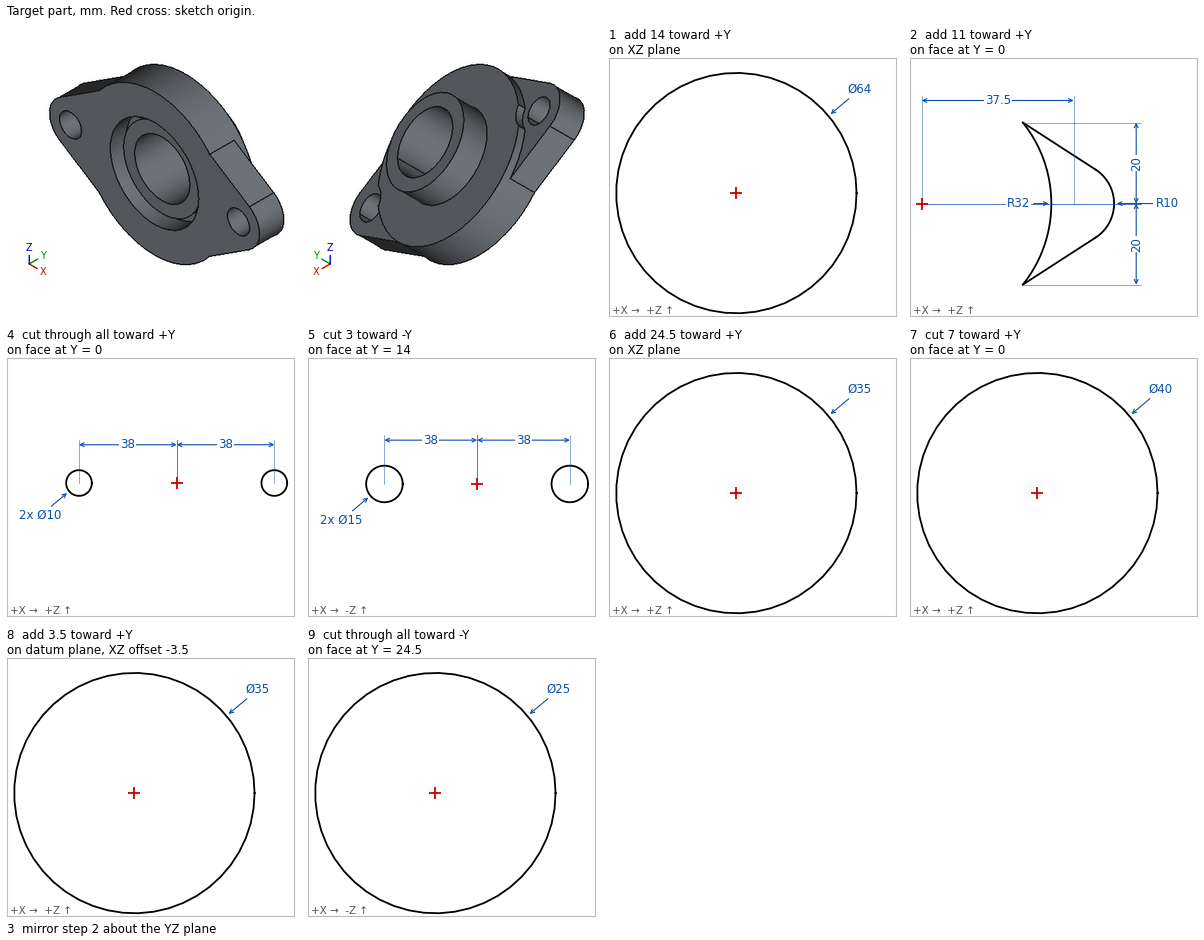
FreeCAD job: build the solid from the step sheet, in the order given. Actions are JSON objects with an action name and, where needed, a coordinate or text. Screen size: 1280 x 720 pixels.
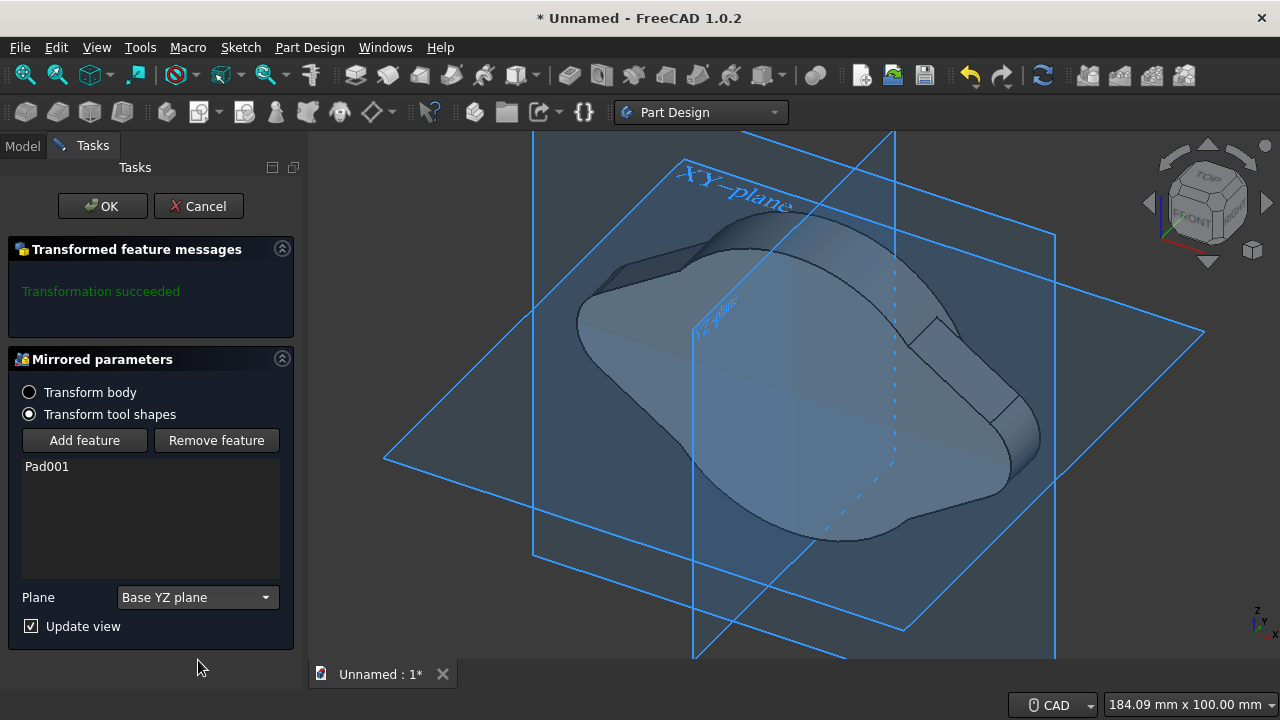
{"action": "left_click", "coordinate": [103, 206]}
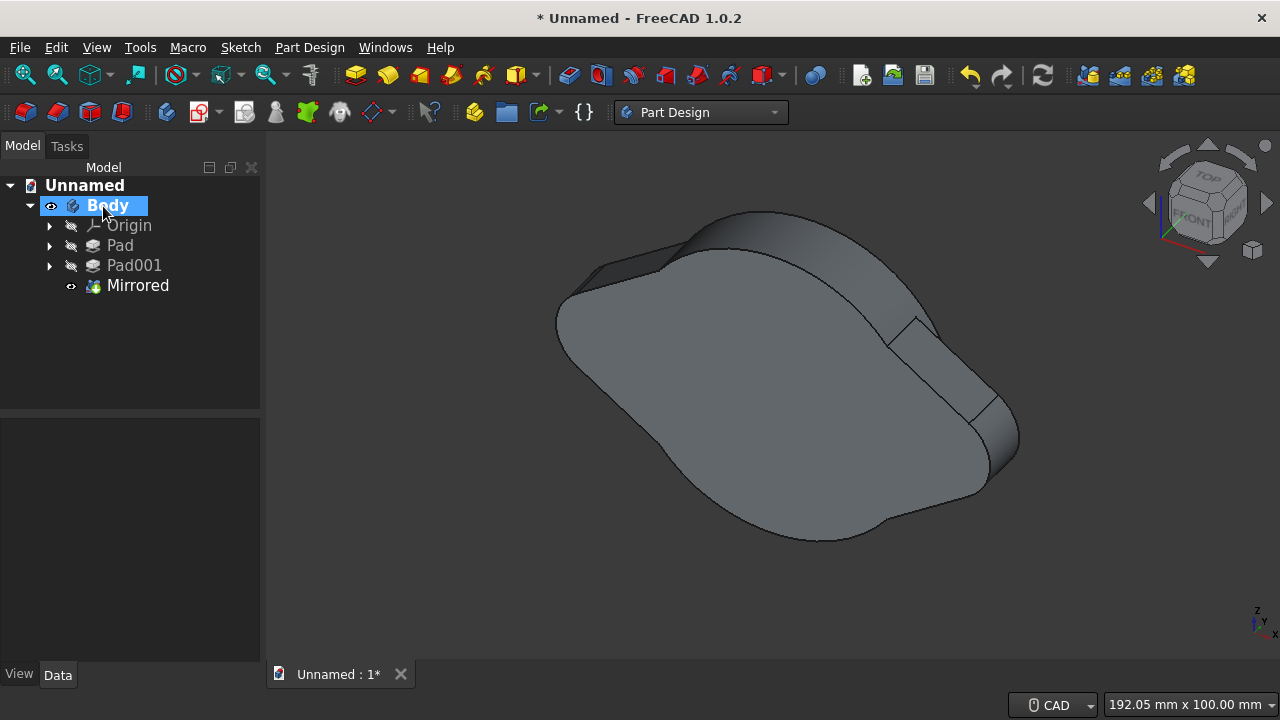
{"action": "left_click", "coordinate": [773, 394]}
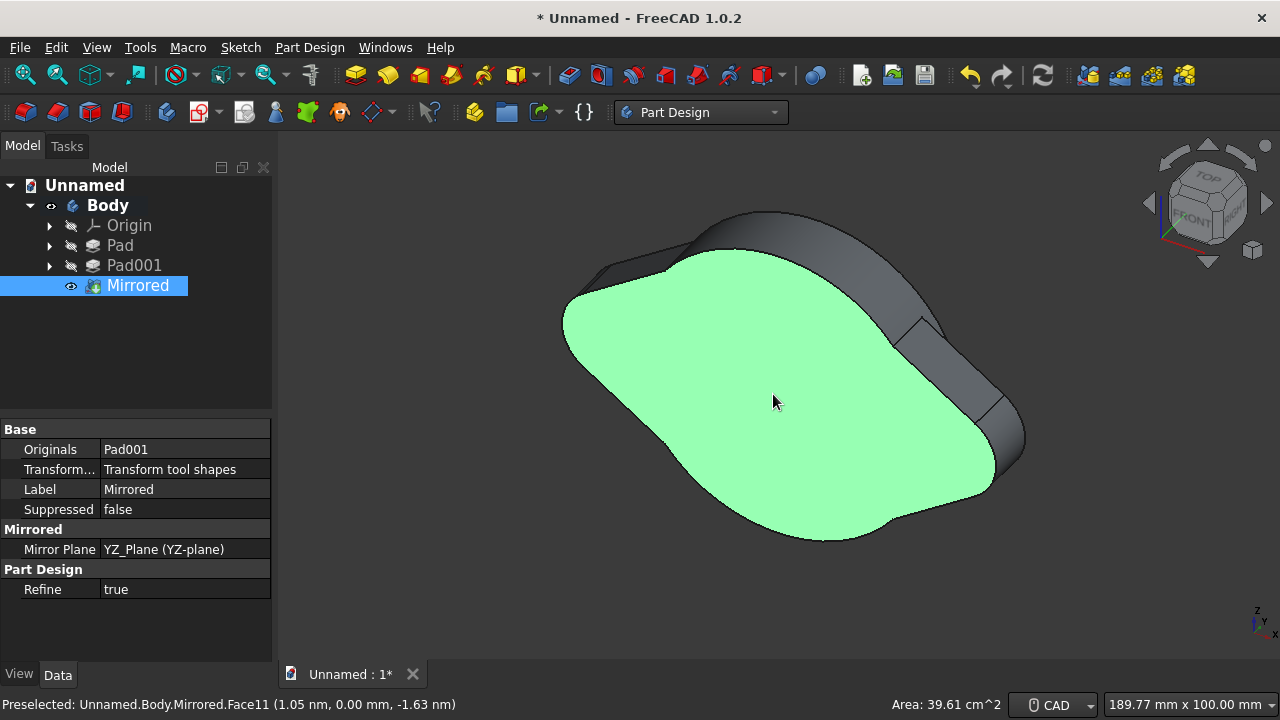
{"action": "left_click", "coordinate": [200, 112]}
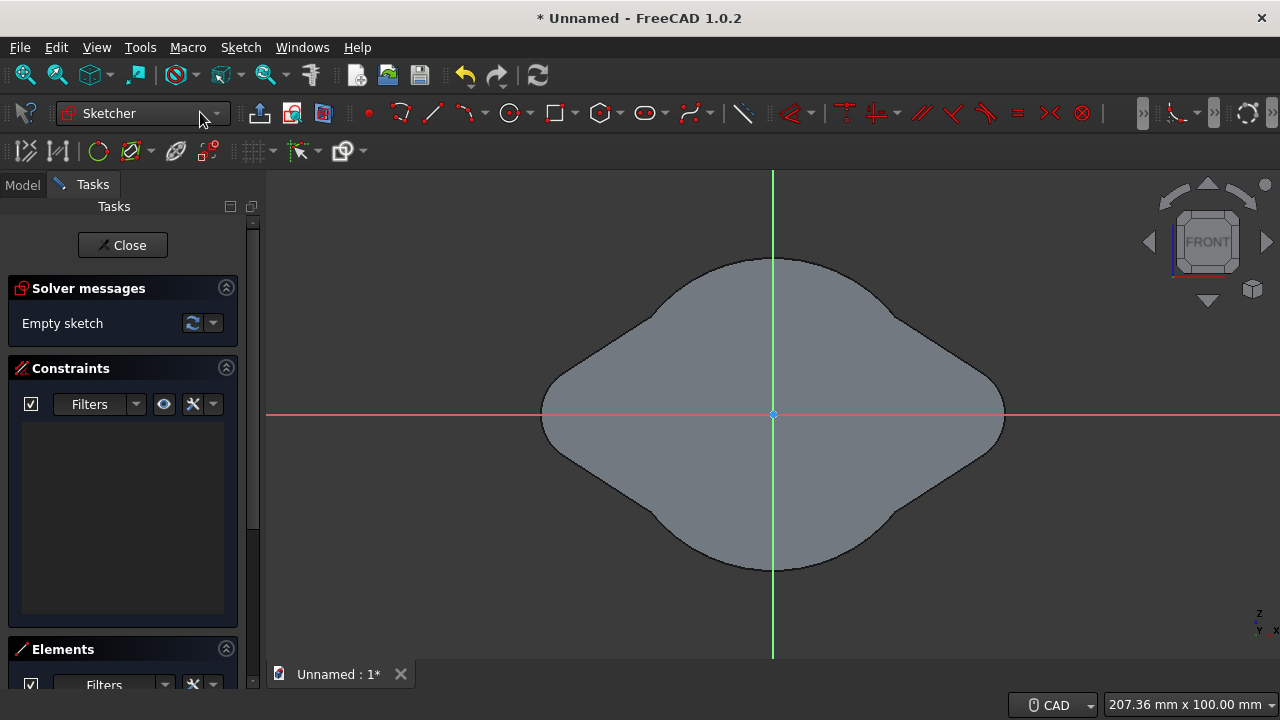
{"action": "scroll", "coordinate": [912, 414], "scroll_direction": "up", "scroll_amount": 2}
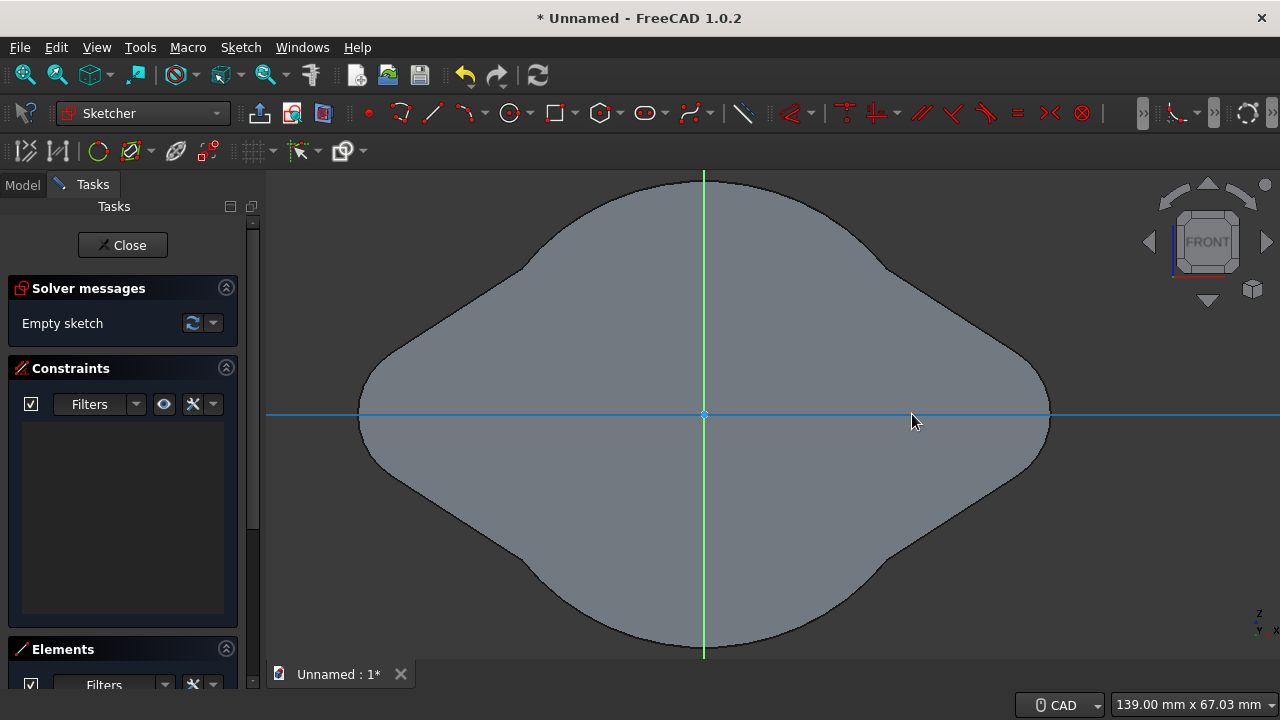
{"action": "key", "text": "g c"}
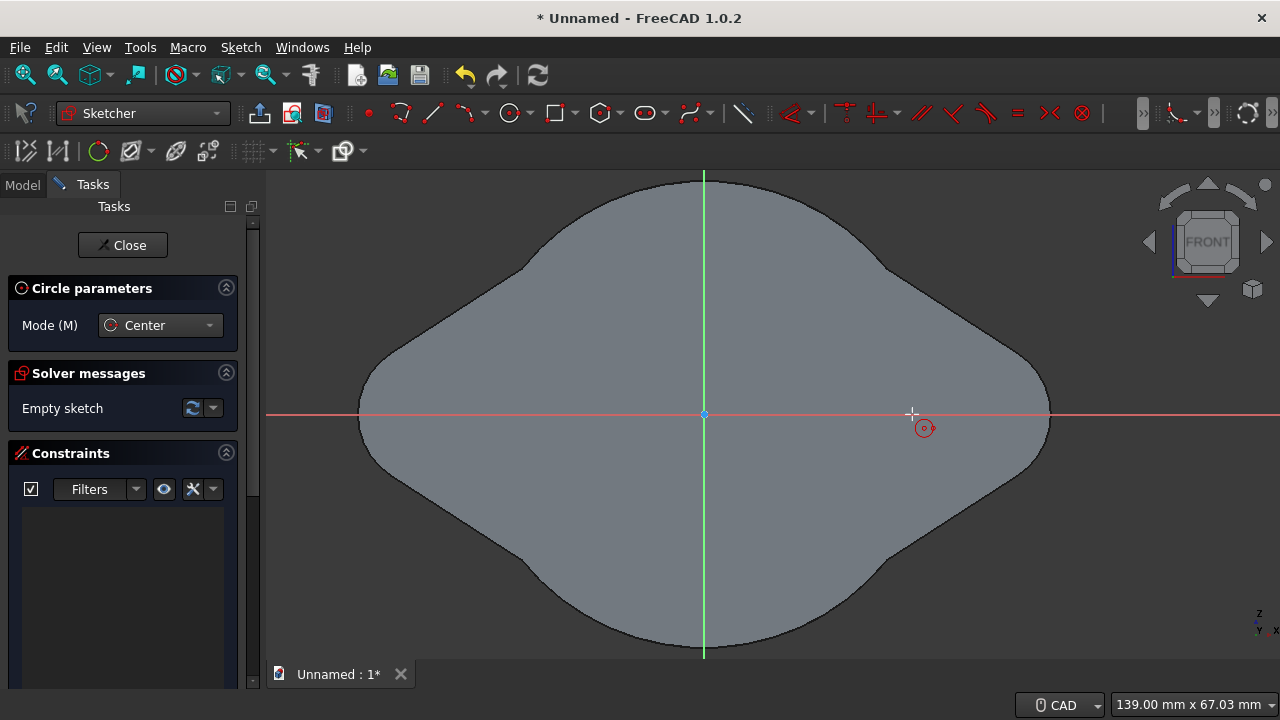
{"action": "left_click", "coordinate": [427, 414]}
{"action": "left_click", "coordinate": [453, 389]}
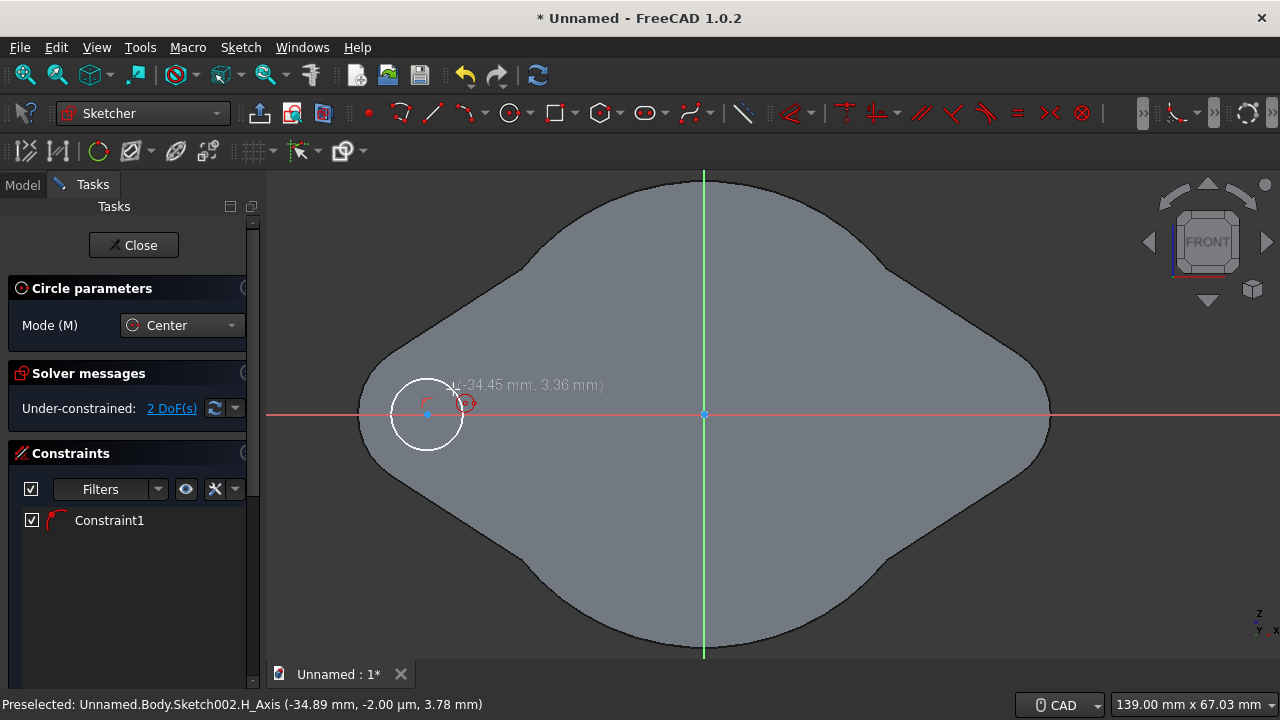
{"action": "left_click", "coordinate": [982, 414]}
{"action": "left_click", "coordinate": [1007, 389]}
{"action": "key", "text": "Escape"}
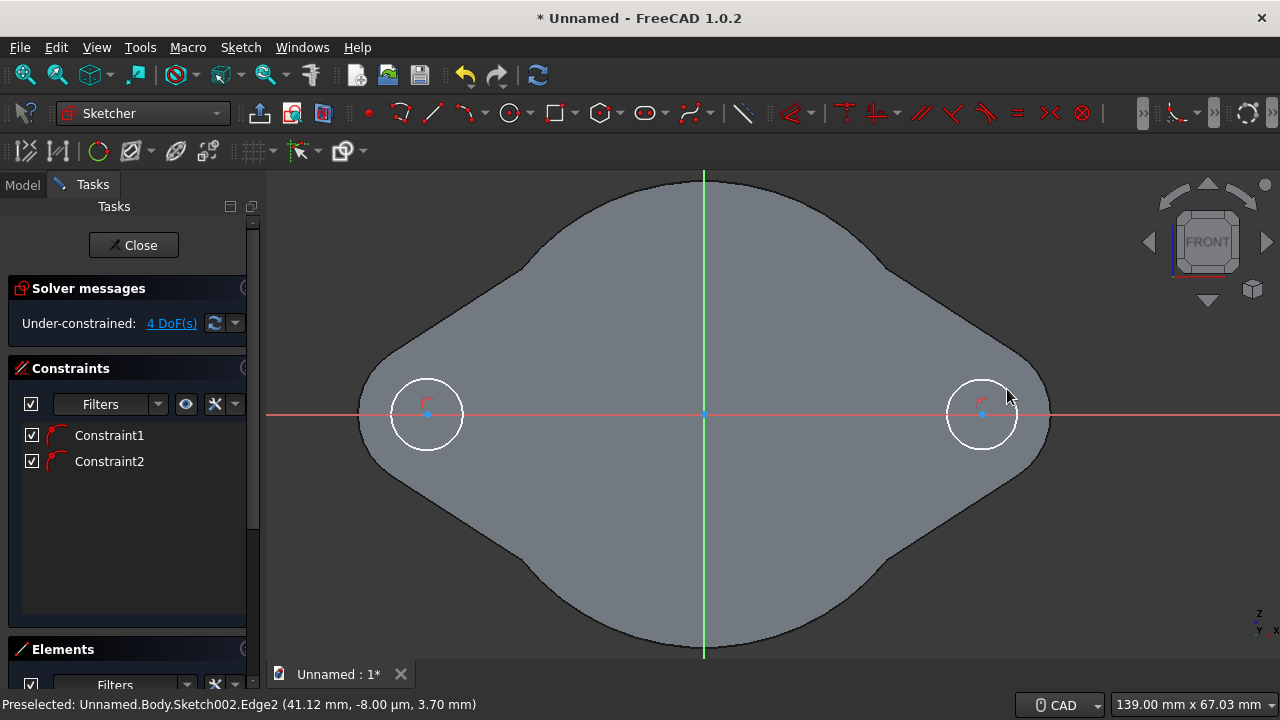
{"action": "left_click", "coordinate": [452, 389]}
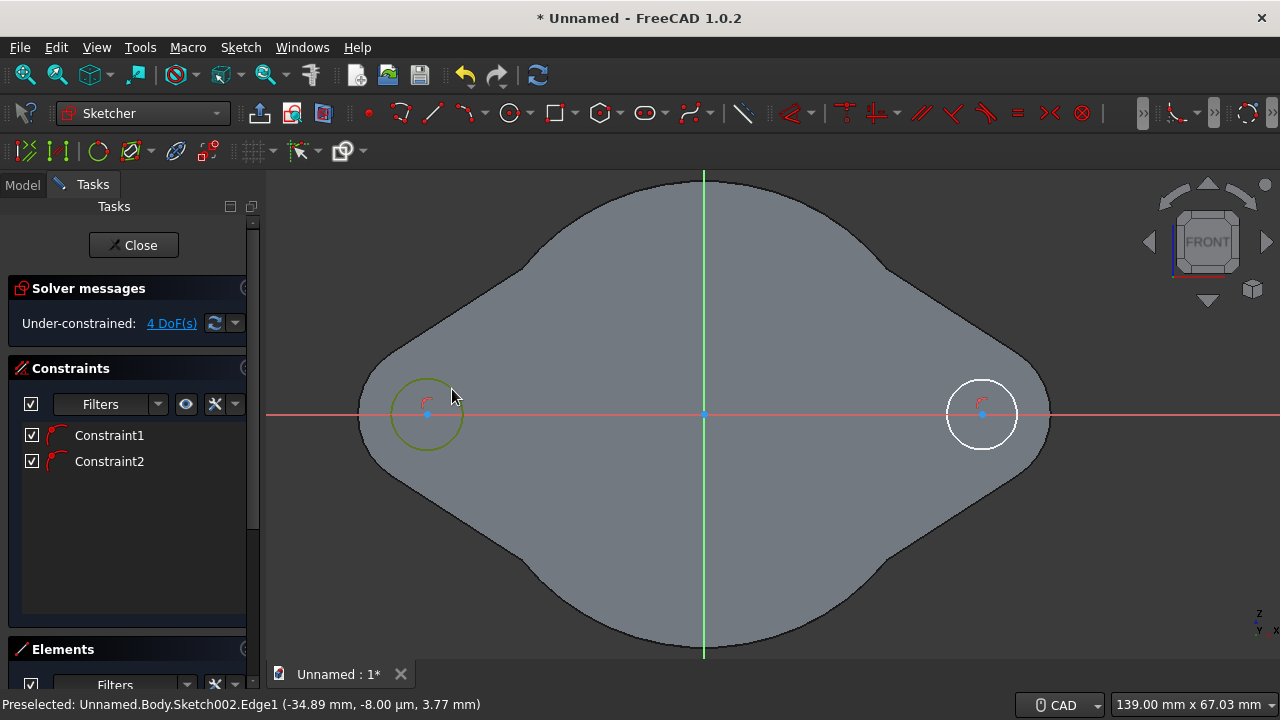
{"action": "left_click", "coordinate": [1007, 390]}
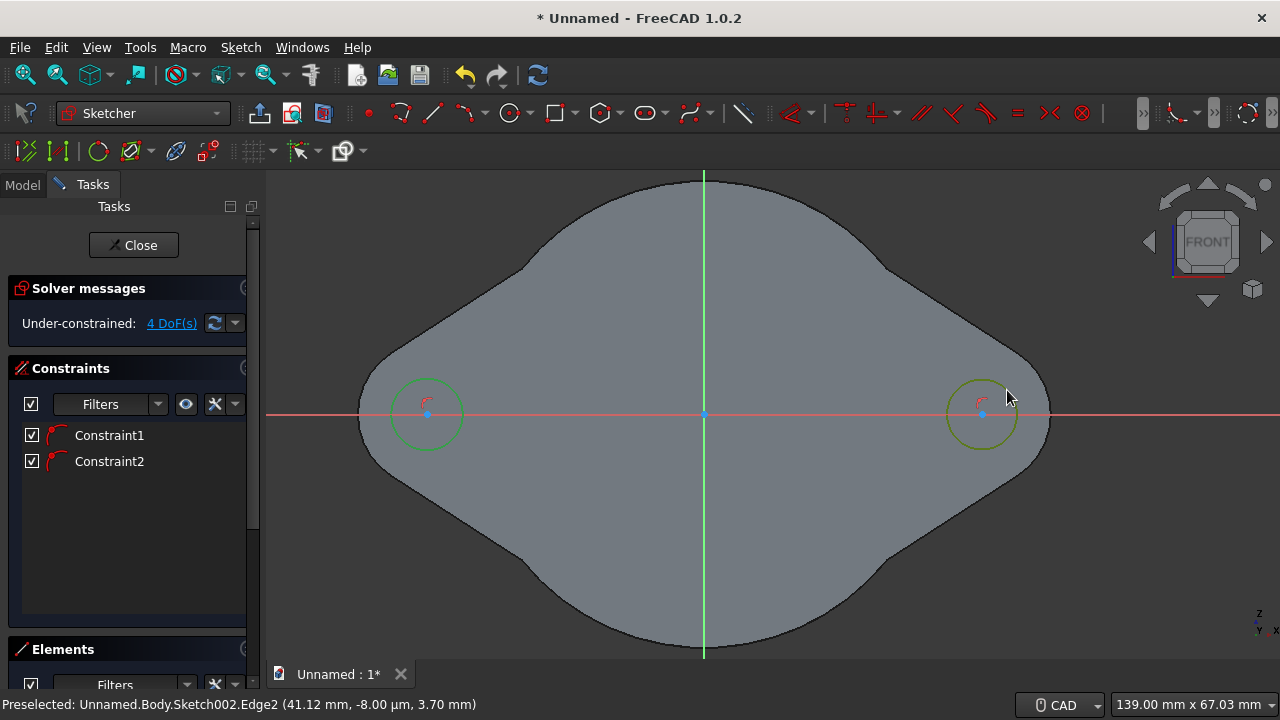
{"action": "left_click", "coordinate": [1018, 114]}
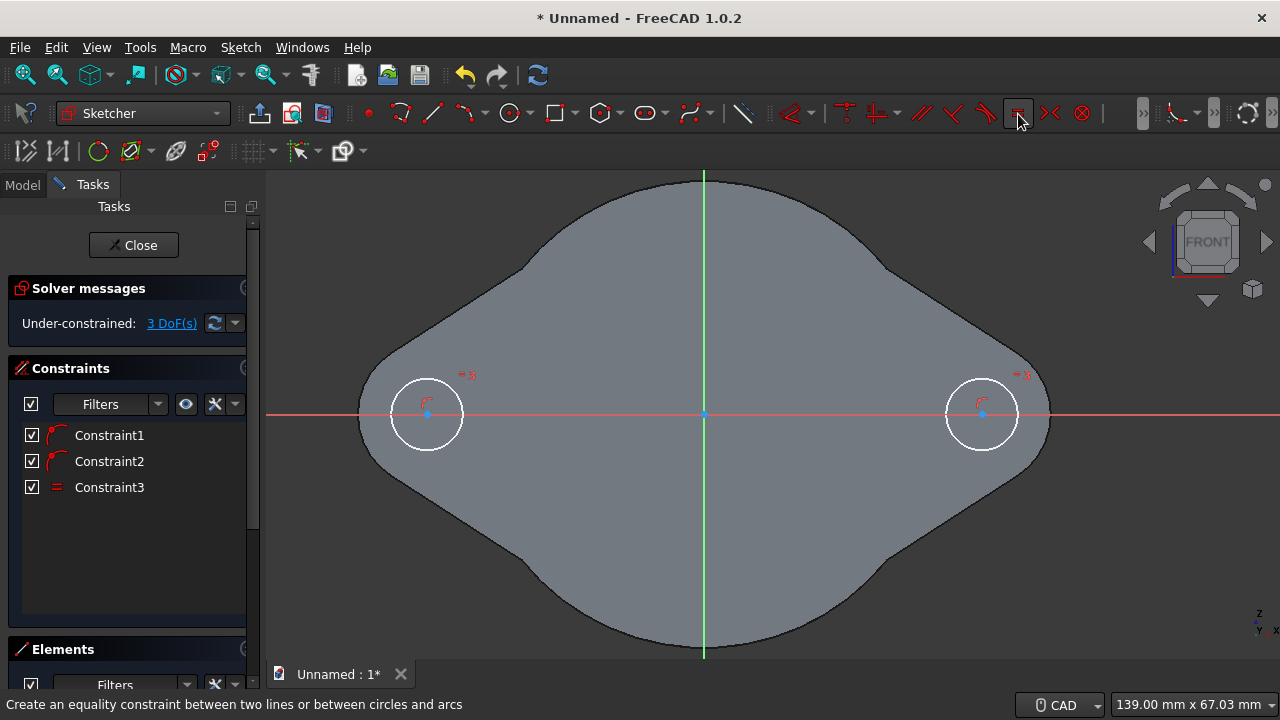
{"action": "left_click", "coordinate": [790, 114]}